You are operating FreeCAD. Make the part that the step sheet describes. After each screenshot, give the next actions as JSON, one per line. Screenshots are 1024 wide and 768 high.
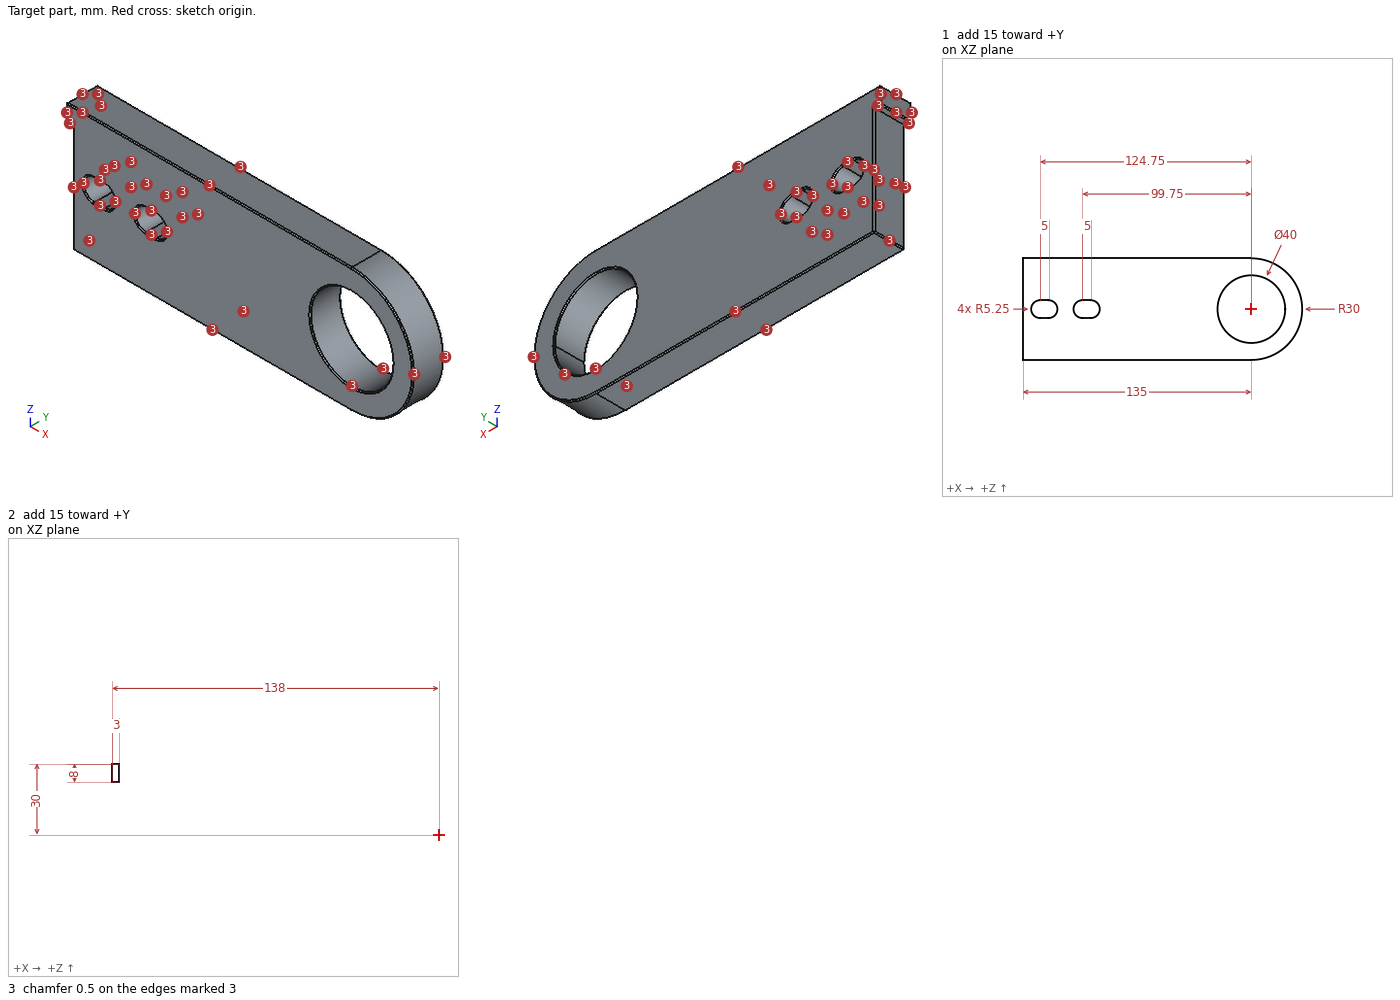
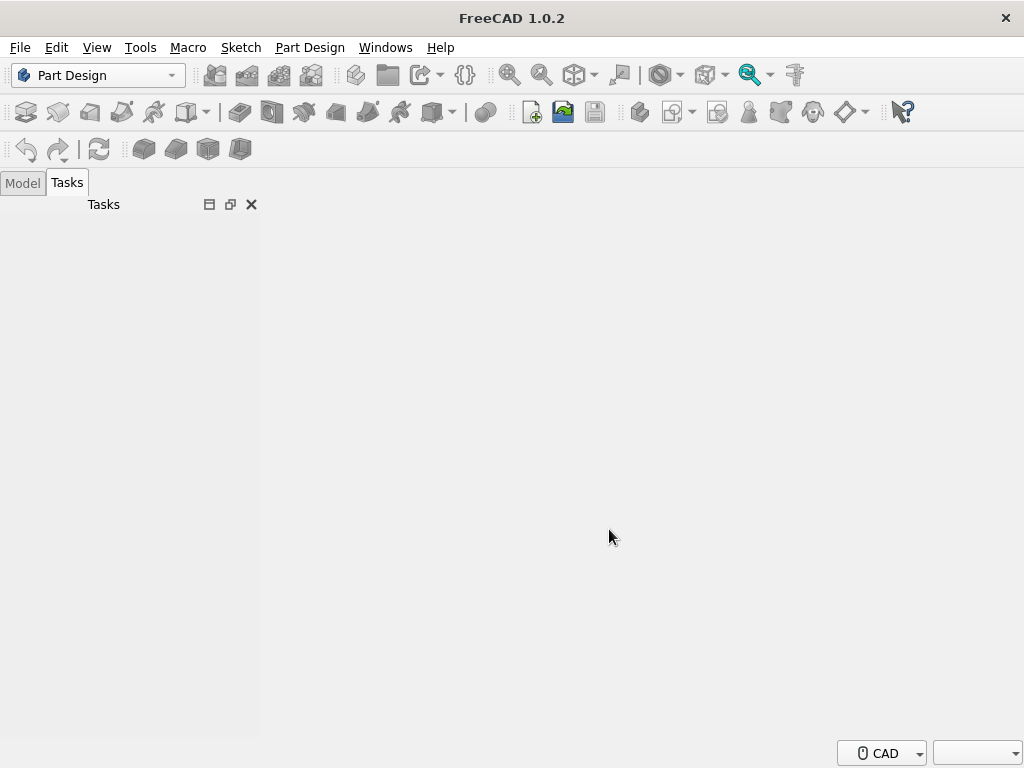
{"action": "left_click", "coordinate": [532, 112]}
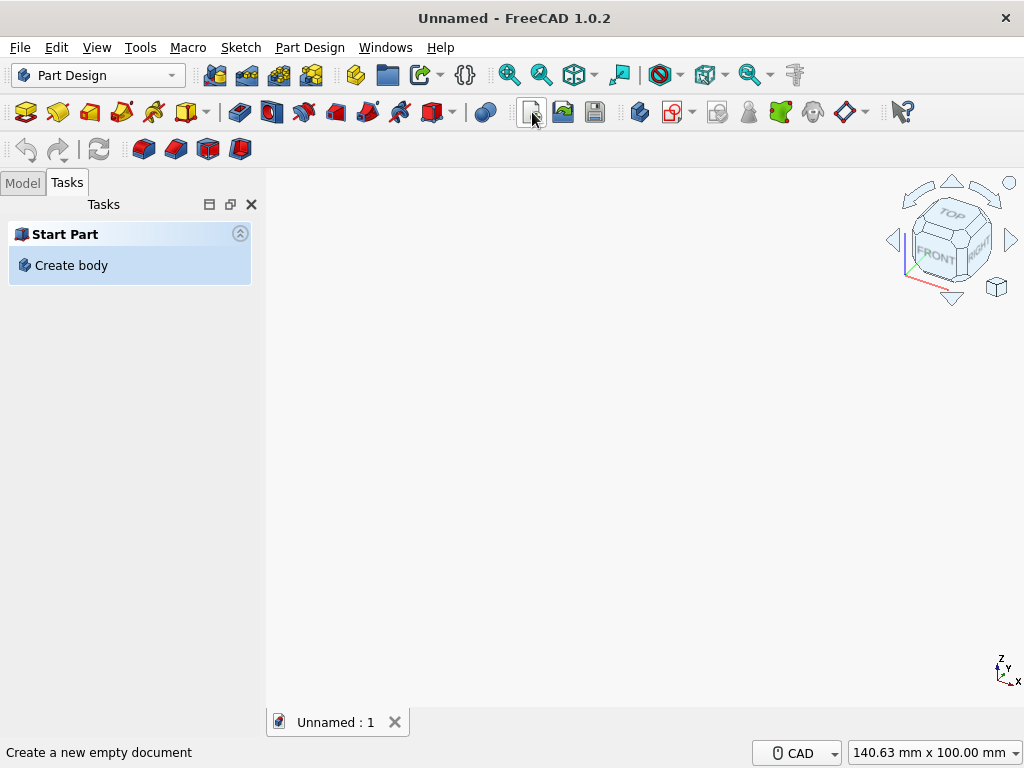
{"action": "left_click", "coordinate": [672, 112]}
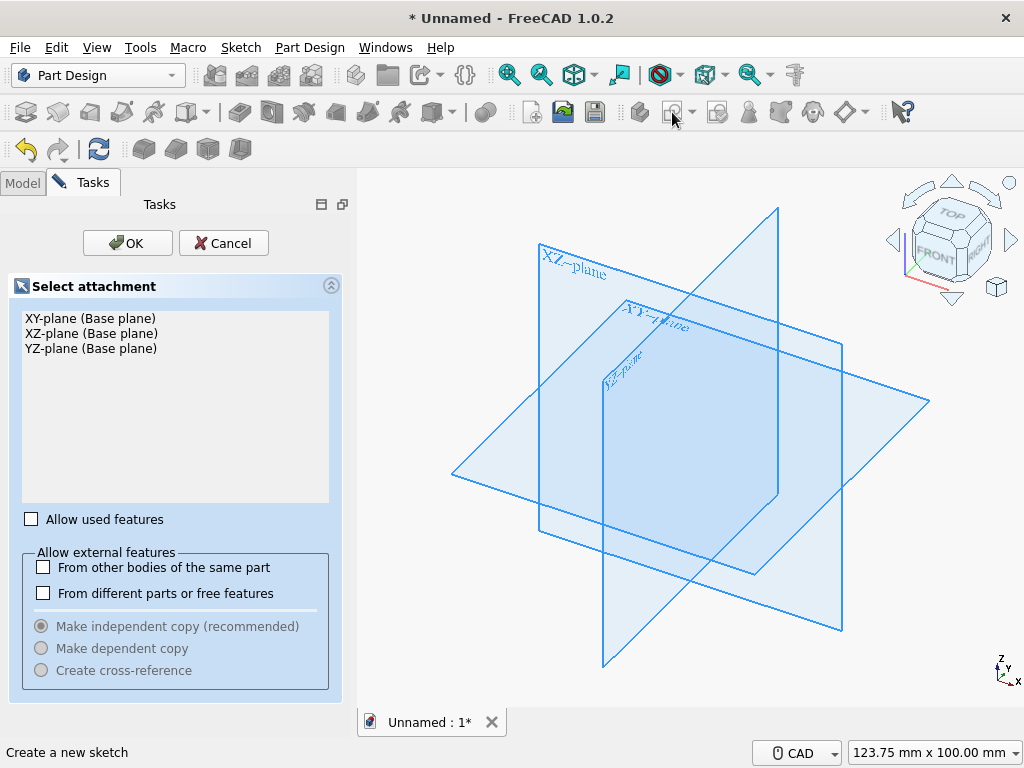
{"action": "left_click", "coordinate": [82, 334]}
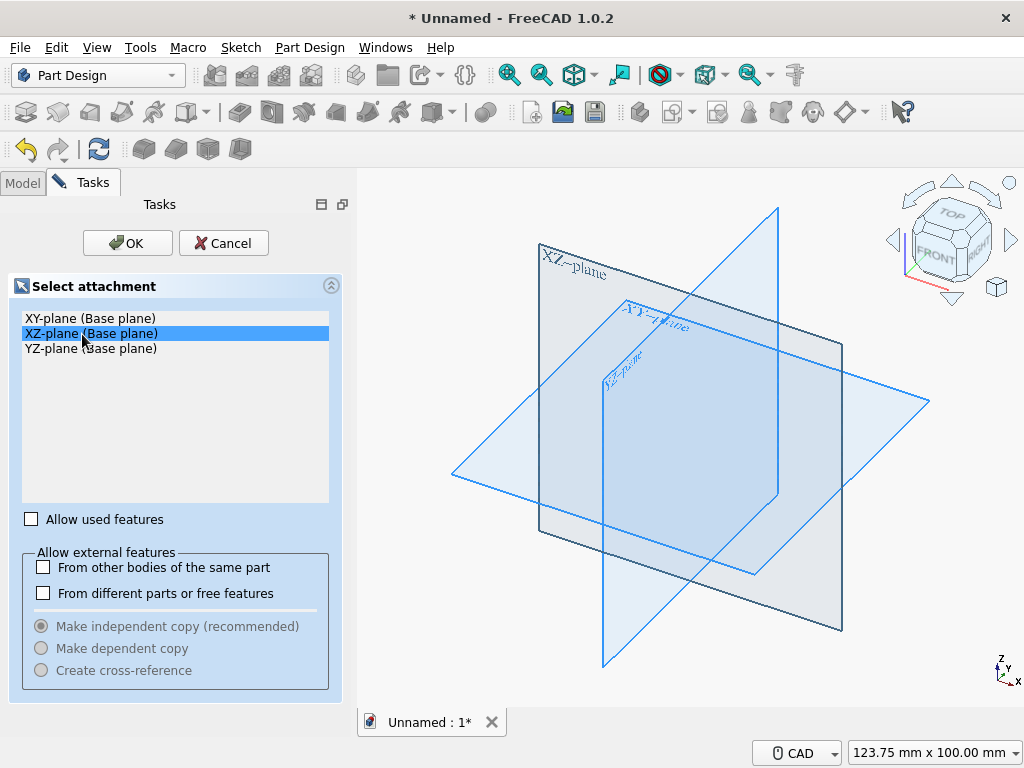
{"action": "left_click", "coordinate": [128, 243]}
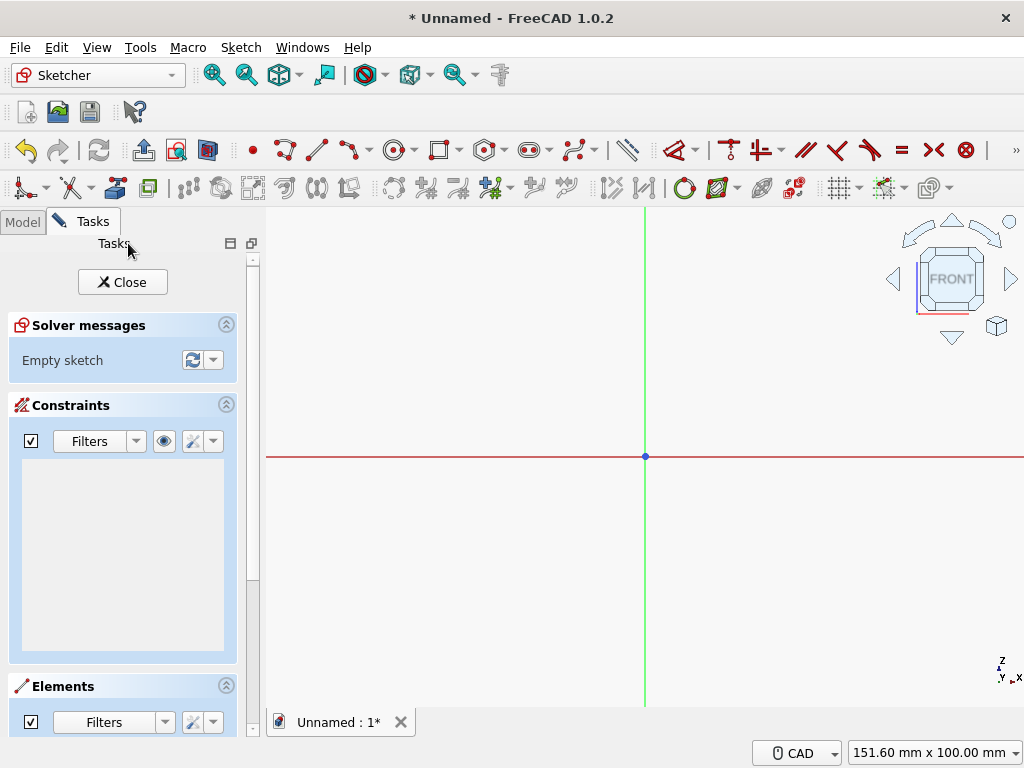
{"action": "scroll", "coordinate": [735, 457], "scroll_direction": "down", "scroll_amount": 4}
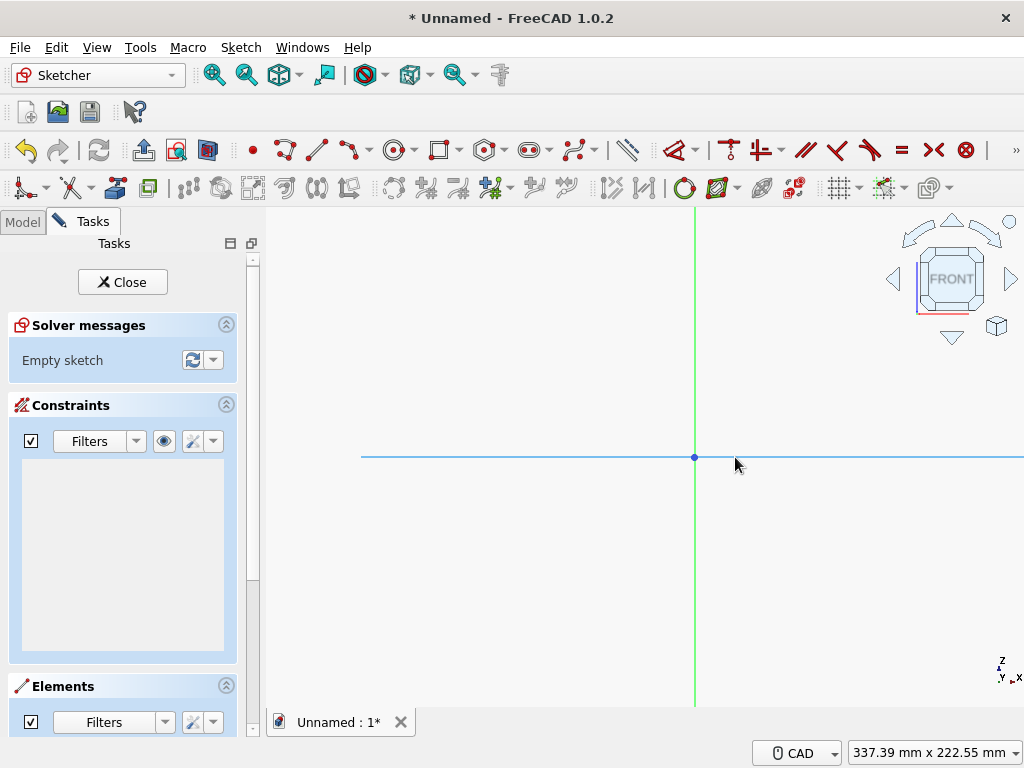
{"action": "left_click", "coordinate": [286, 150]}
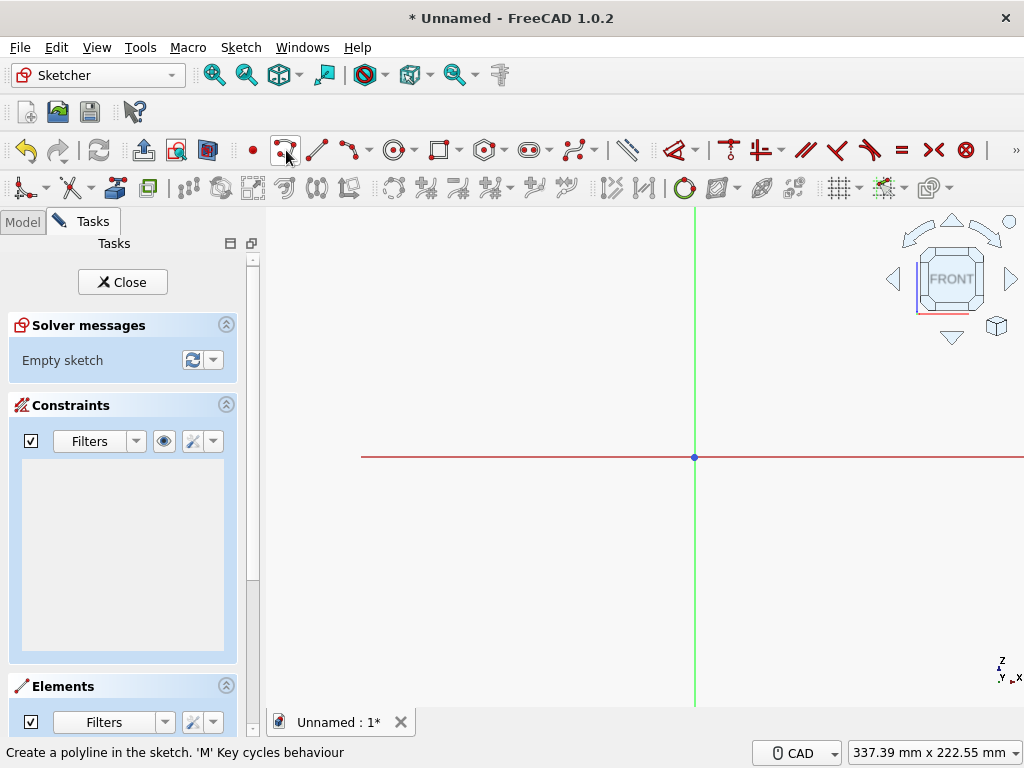
{"action": "left_click", "coordinate": [695, 525]}
{"action": "left_click", "coordinate": [392, 525]}
{"action": "left_click", "coordinate": [392, 390]}
{"action": "left_click", "coordinate": [695, 390]}
{"action": "right_click", "coordinate": [695, 390]}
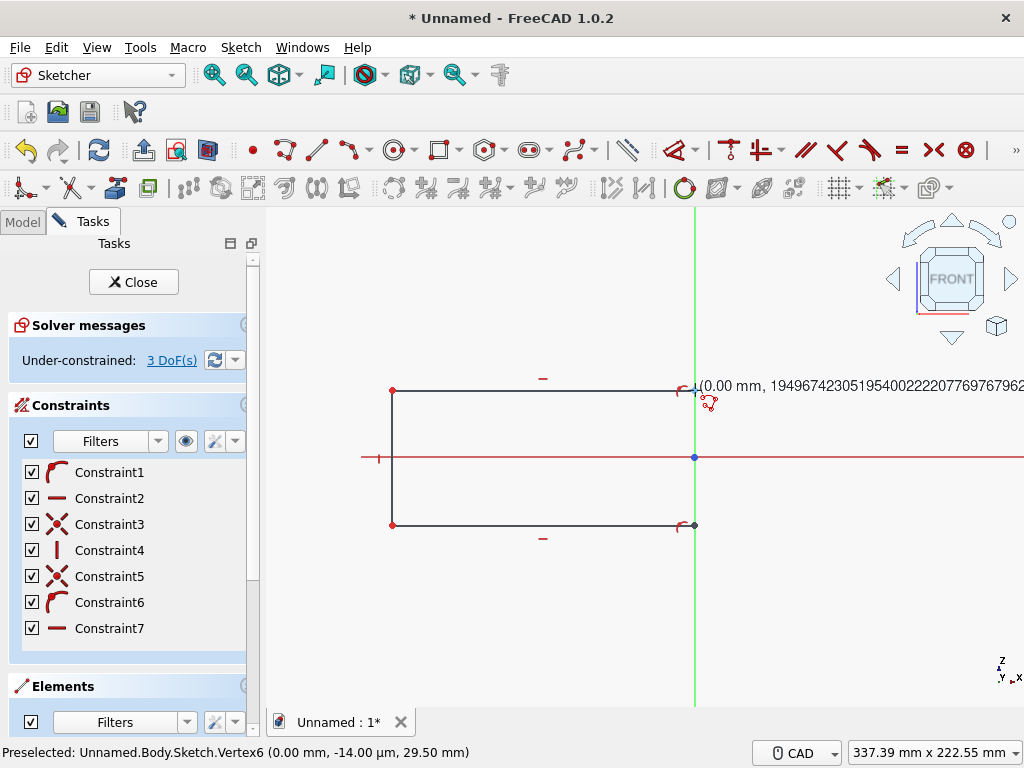
{"action": "left_click", "coordinate": [350, 150]}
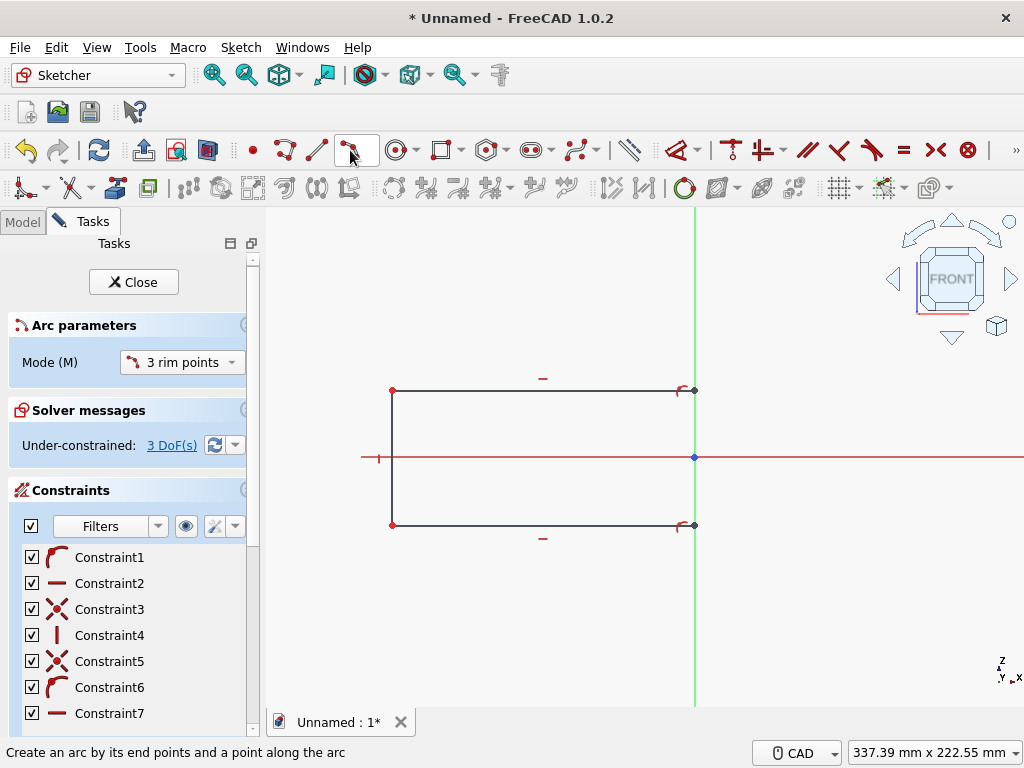
{"action": "left_click", "coordinate": [695, 391]}
{"action": "left_click", "coordinate": [695, 526]}
{"action": "left_click", "coordinate": [759, 478]}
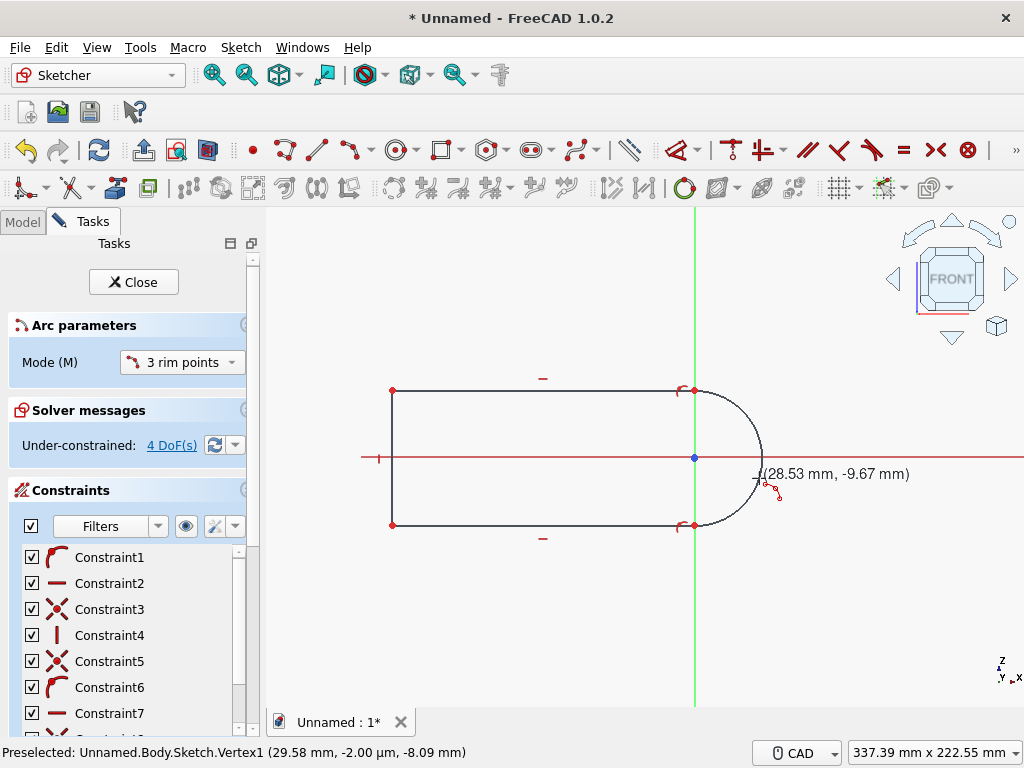
{"action": "left_click", "coordinate": [532, 150]}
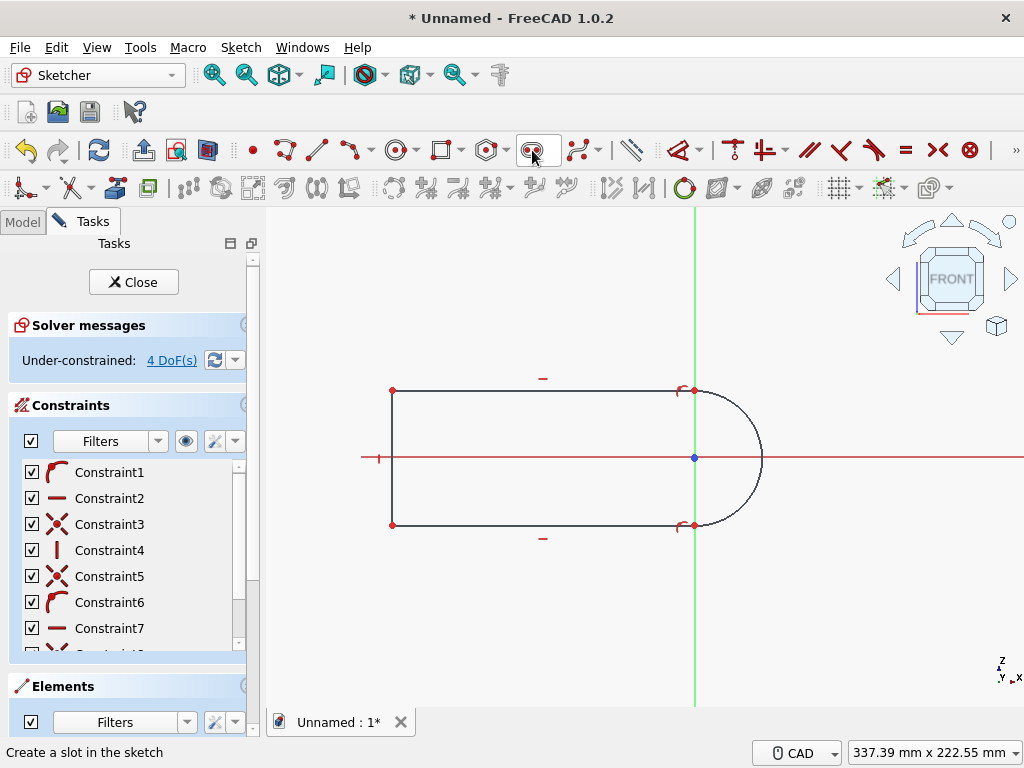
{"action": "scroll", "coordinate": [415, 457], "scroll_direction": "up", "scroll_amount": 4}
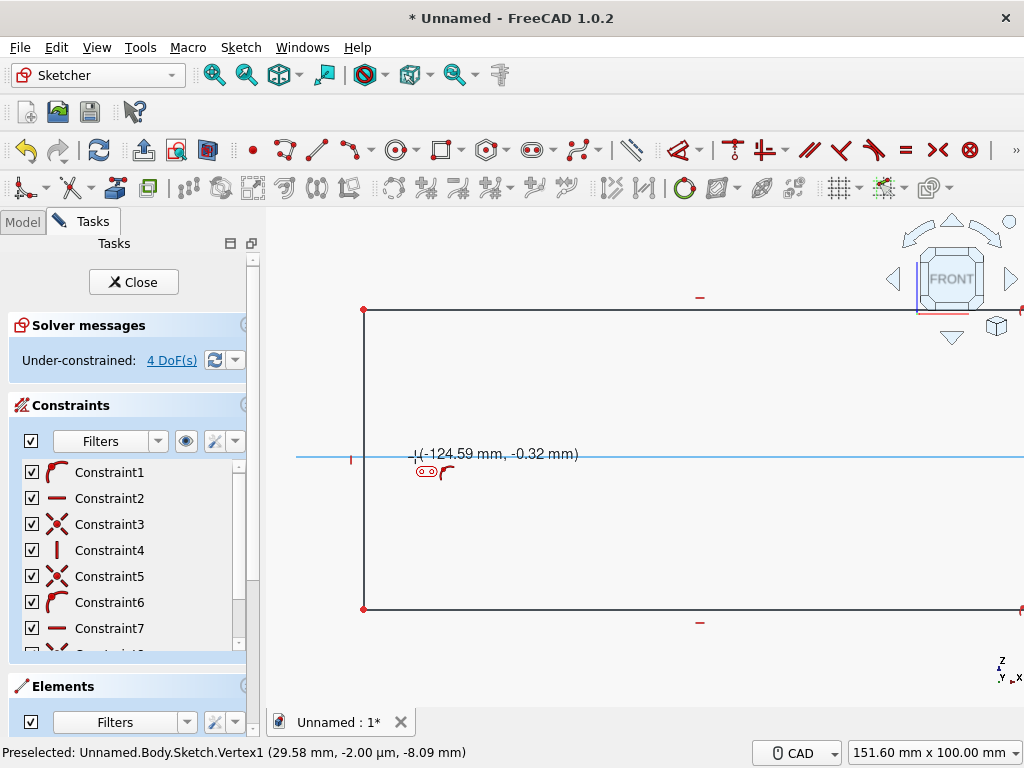
{"action": "left_click", "coordinate": [414, 457]}